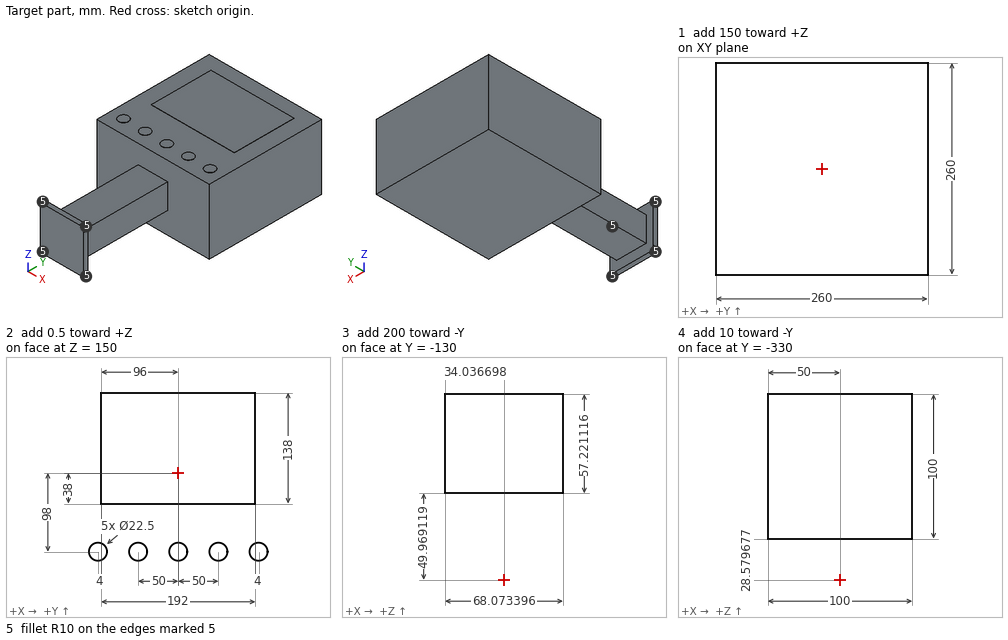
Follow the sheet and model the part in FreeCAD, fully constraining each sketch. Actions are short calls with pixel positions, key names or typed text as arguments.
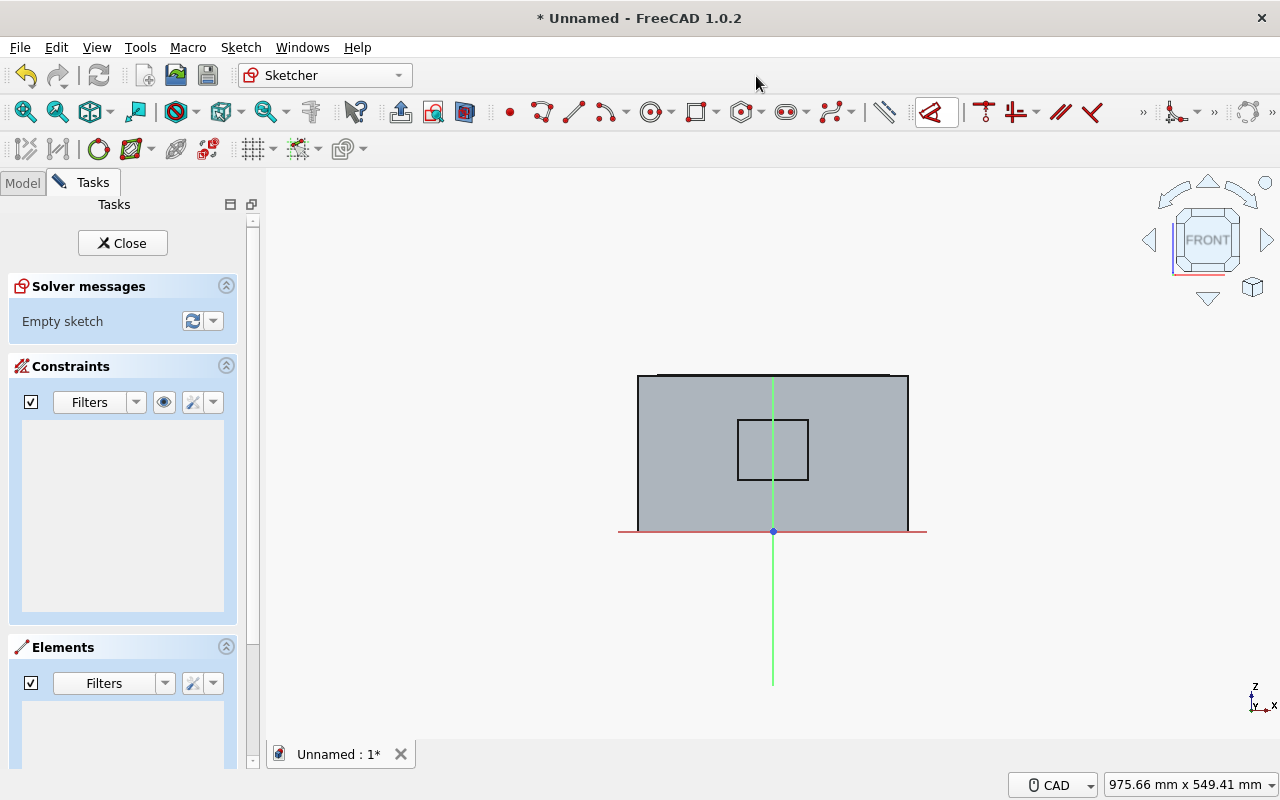
scroll(813, 472, up, 5)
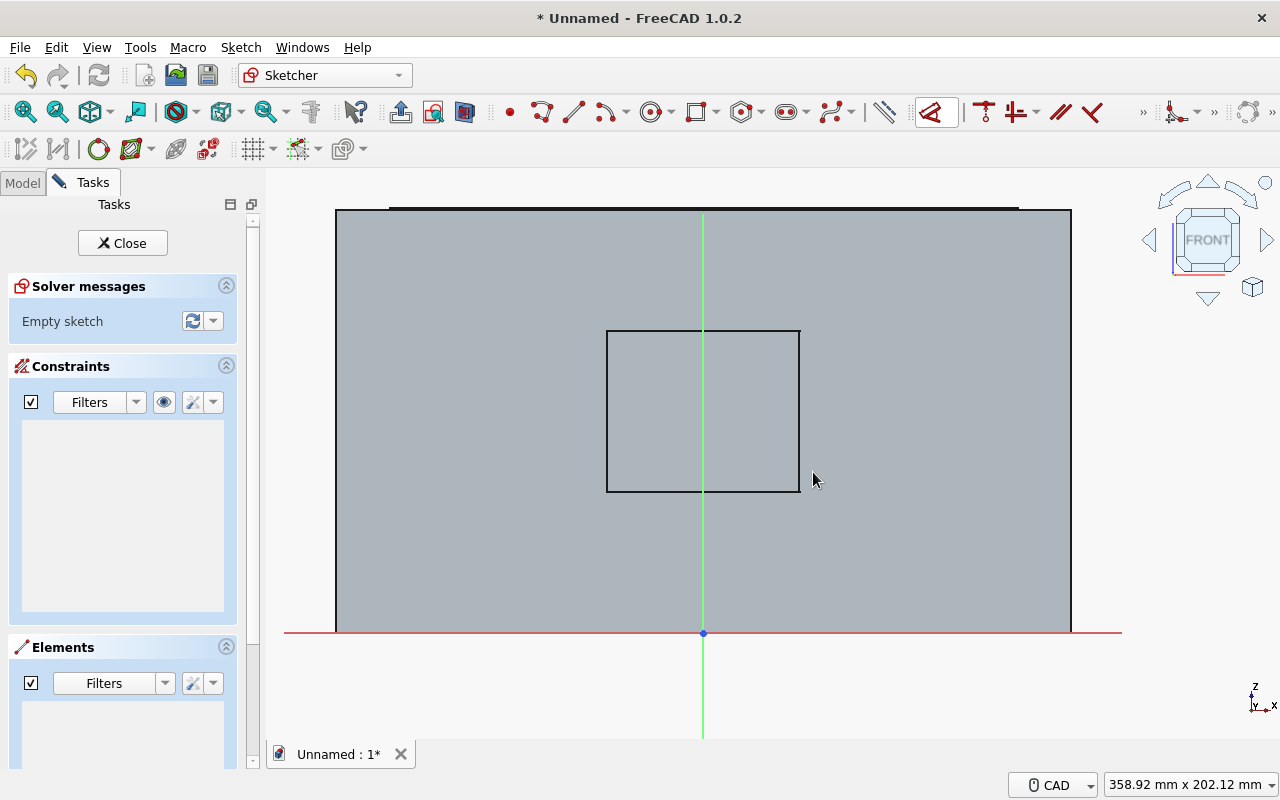
key(g)
key(r)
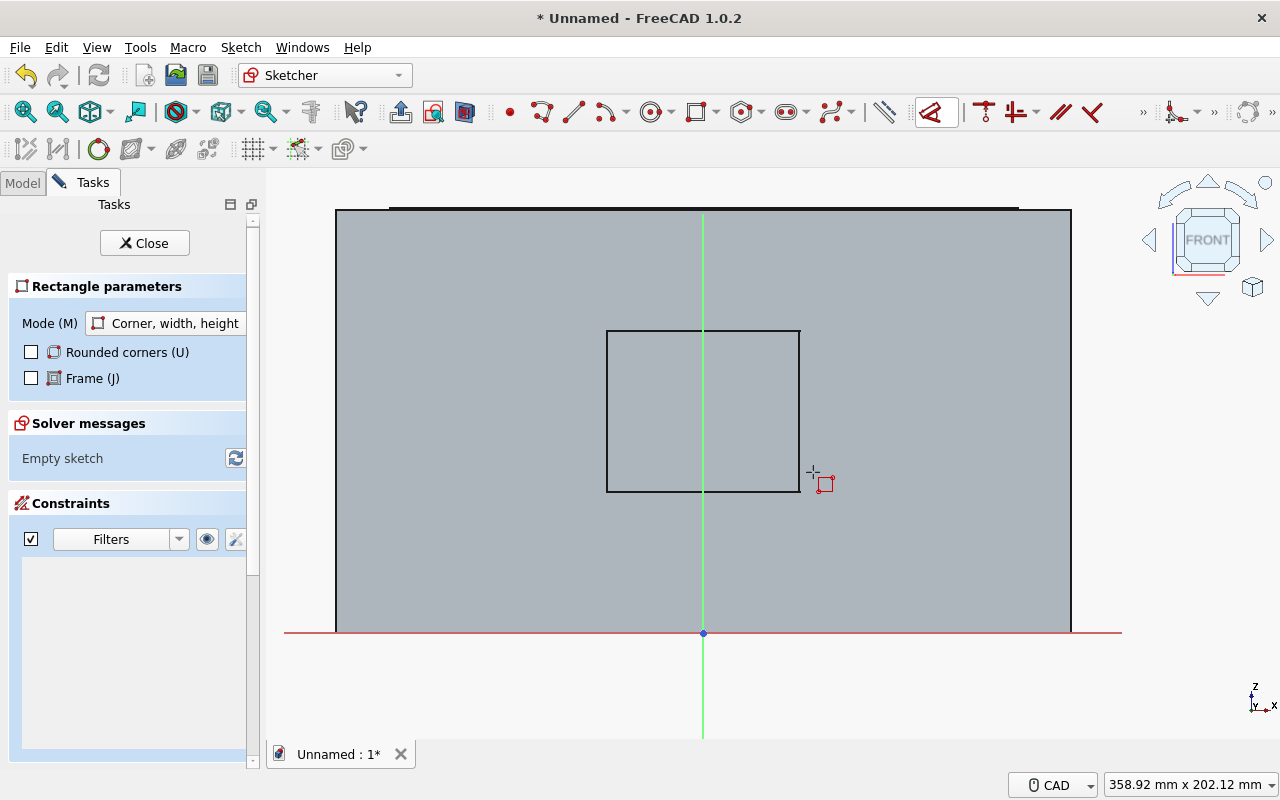
click(562, 270)
move(845, 553)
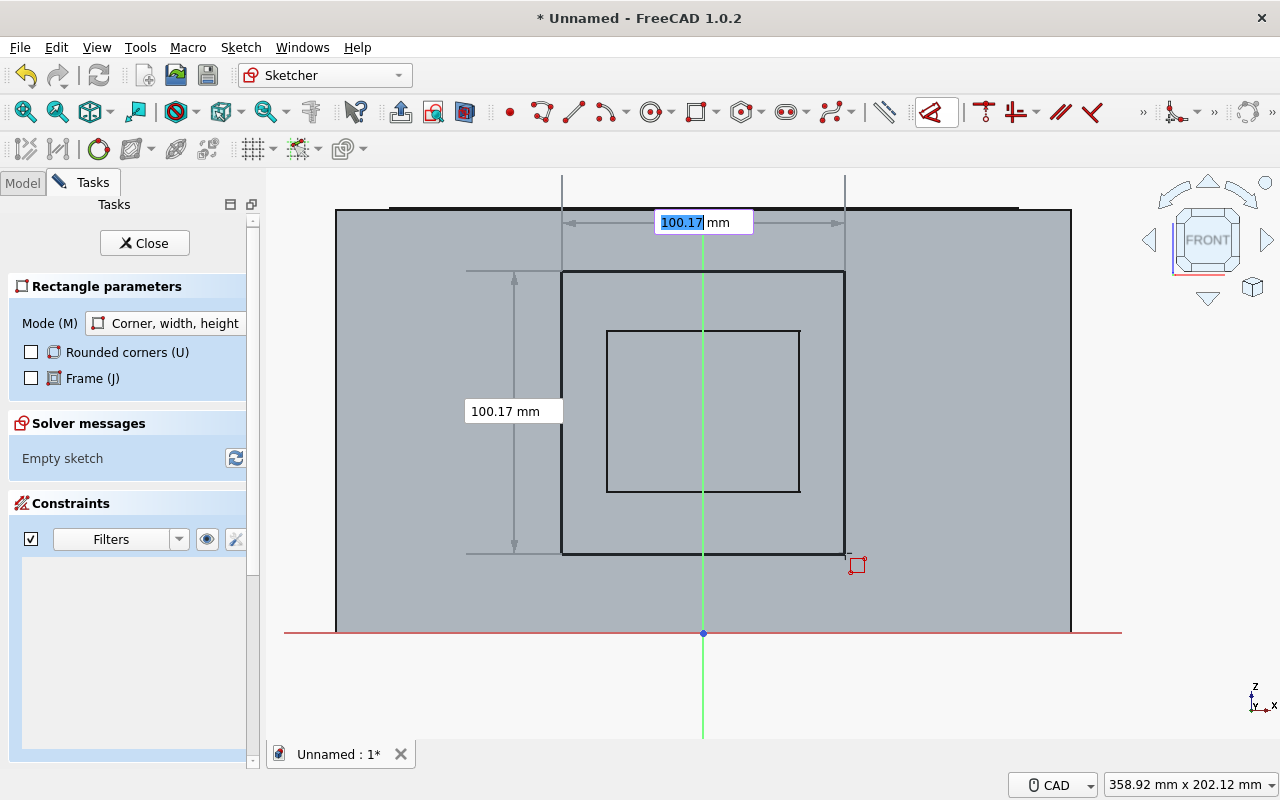
text(100)
key(Tab)
text(100)
key(Return)
key(Escape)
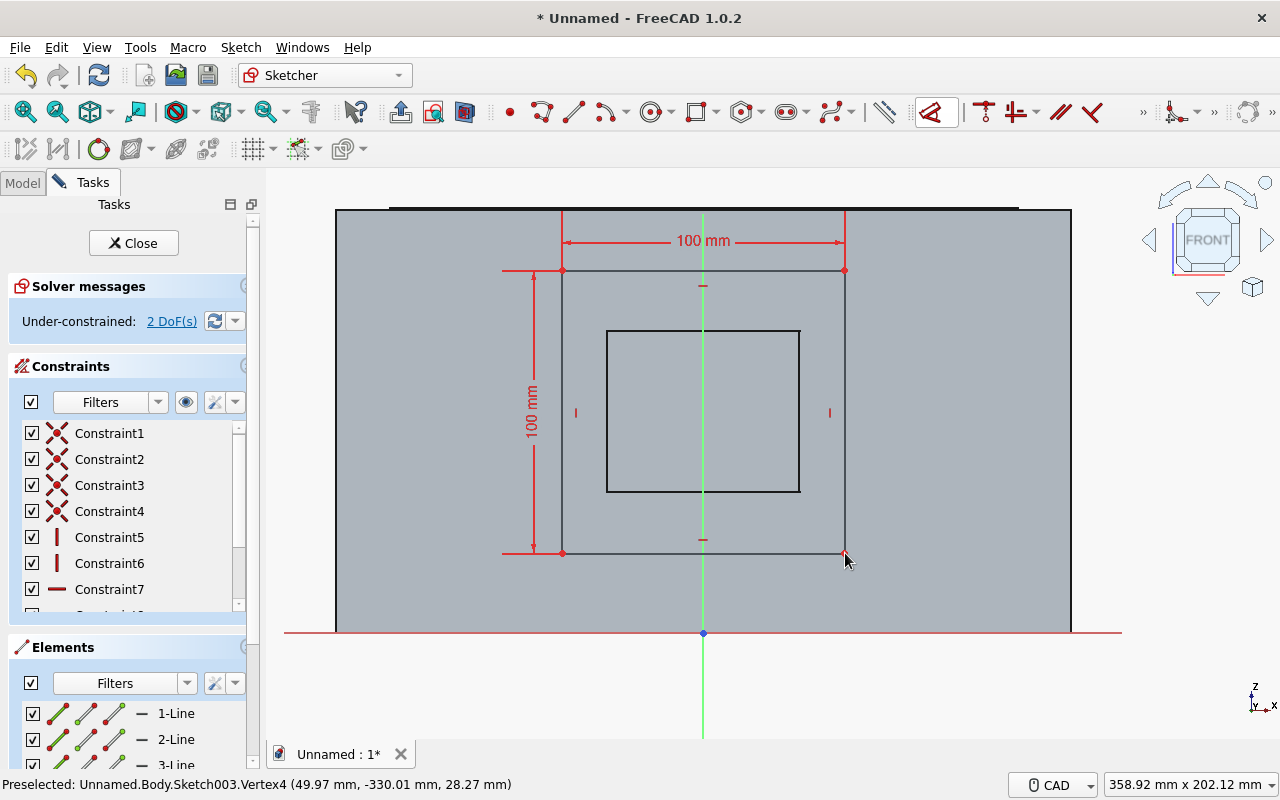
click(562, 271)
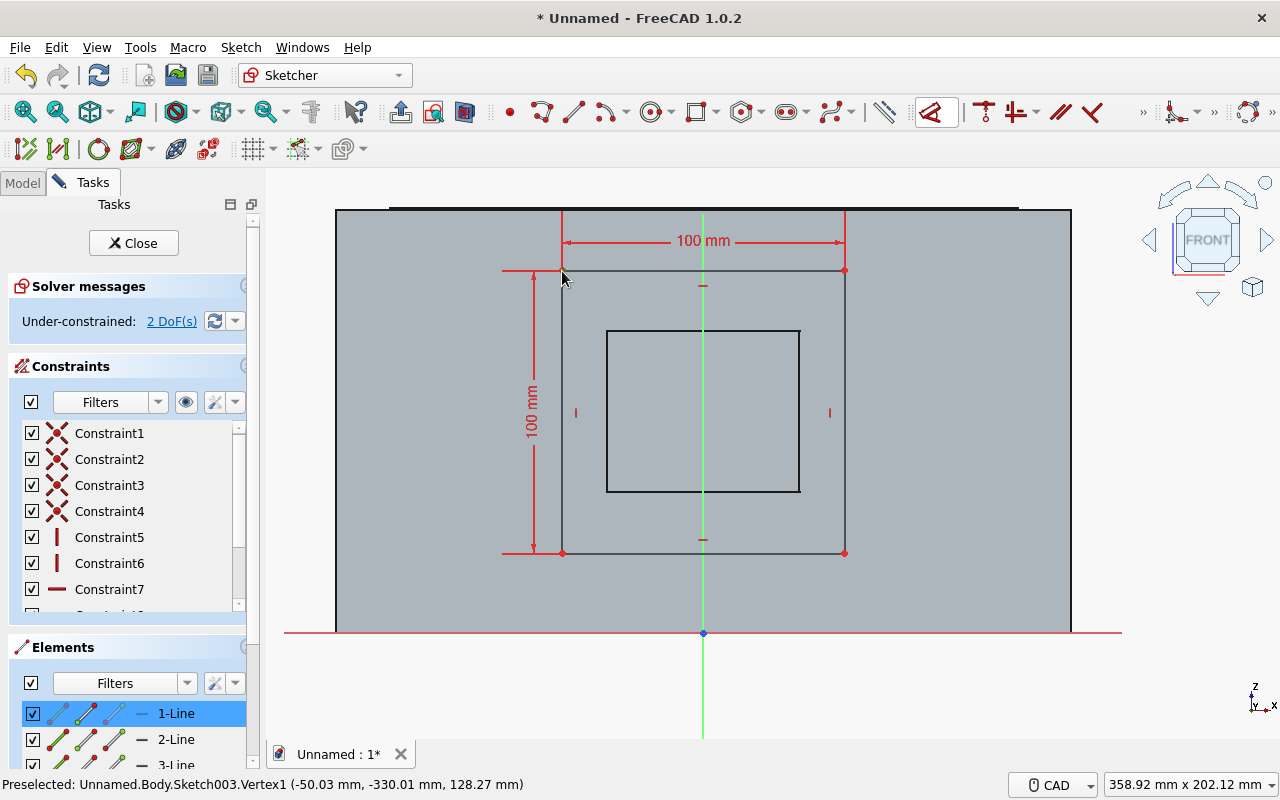
key(l)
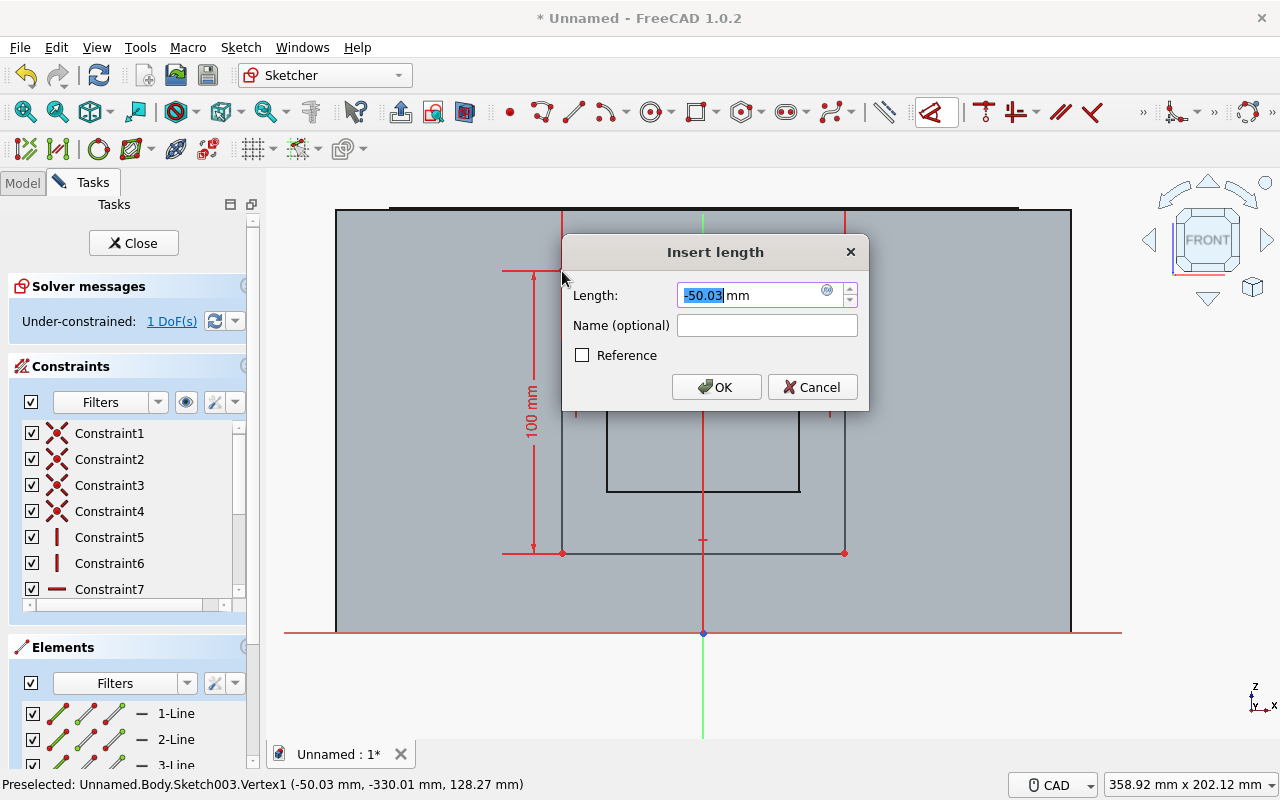
text(-50)
key(Return)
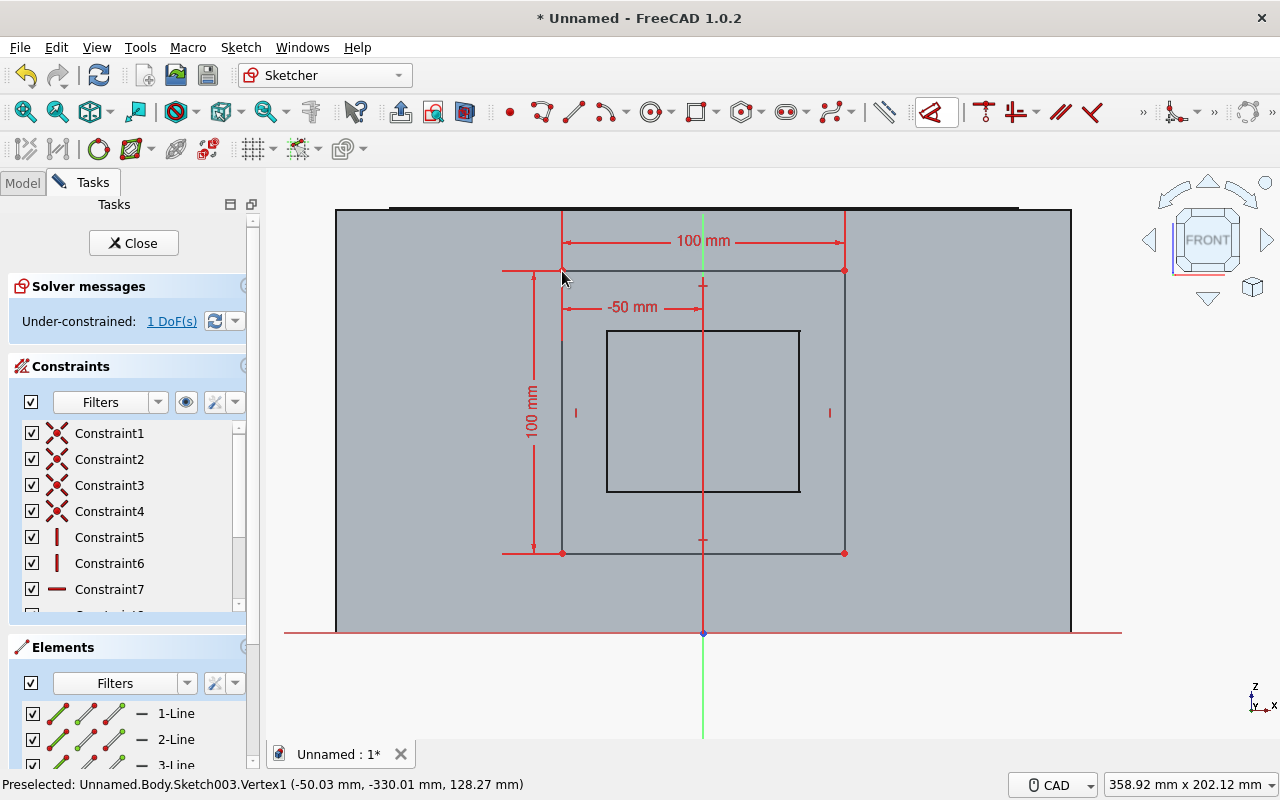
click(562, 554)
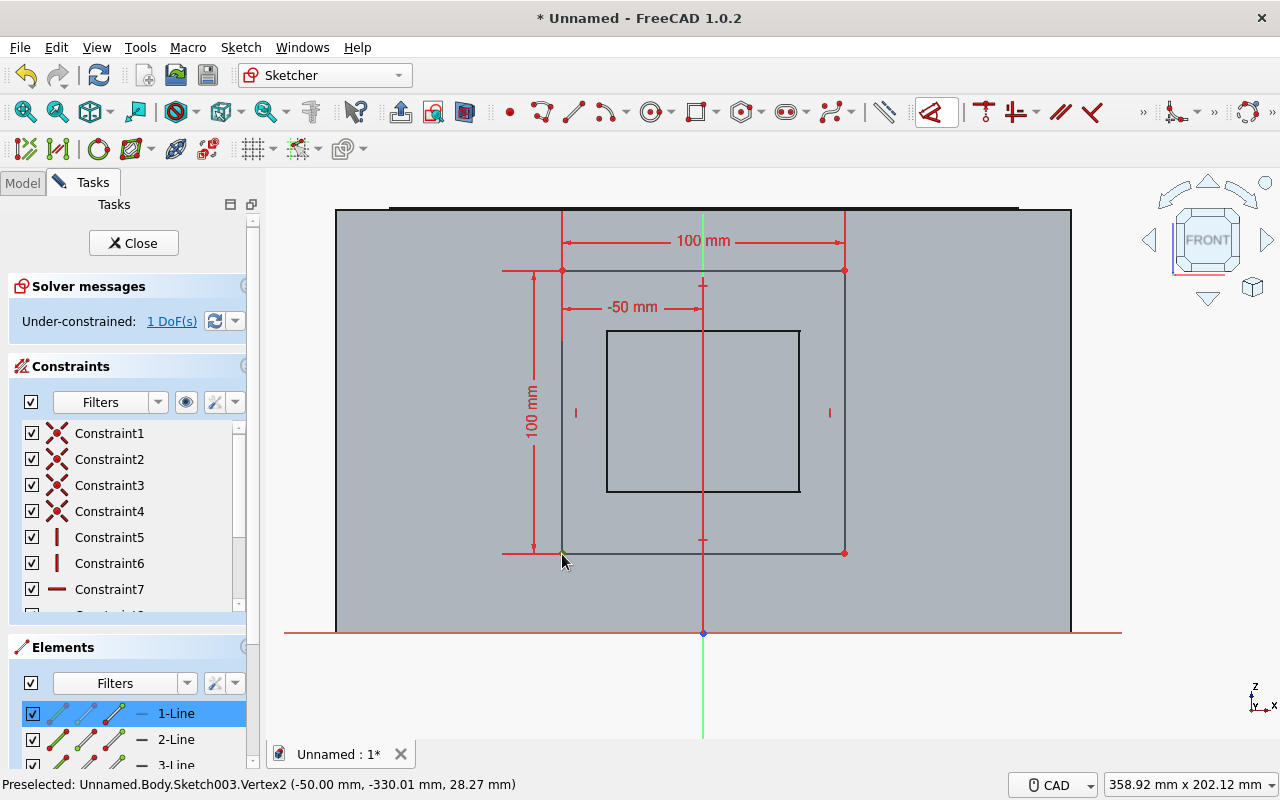
click(952, 112)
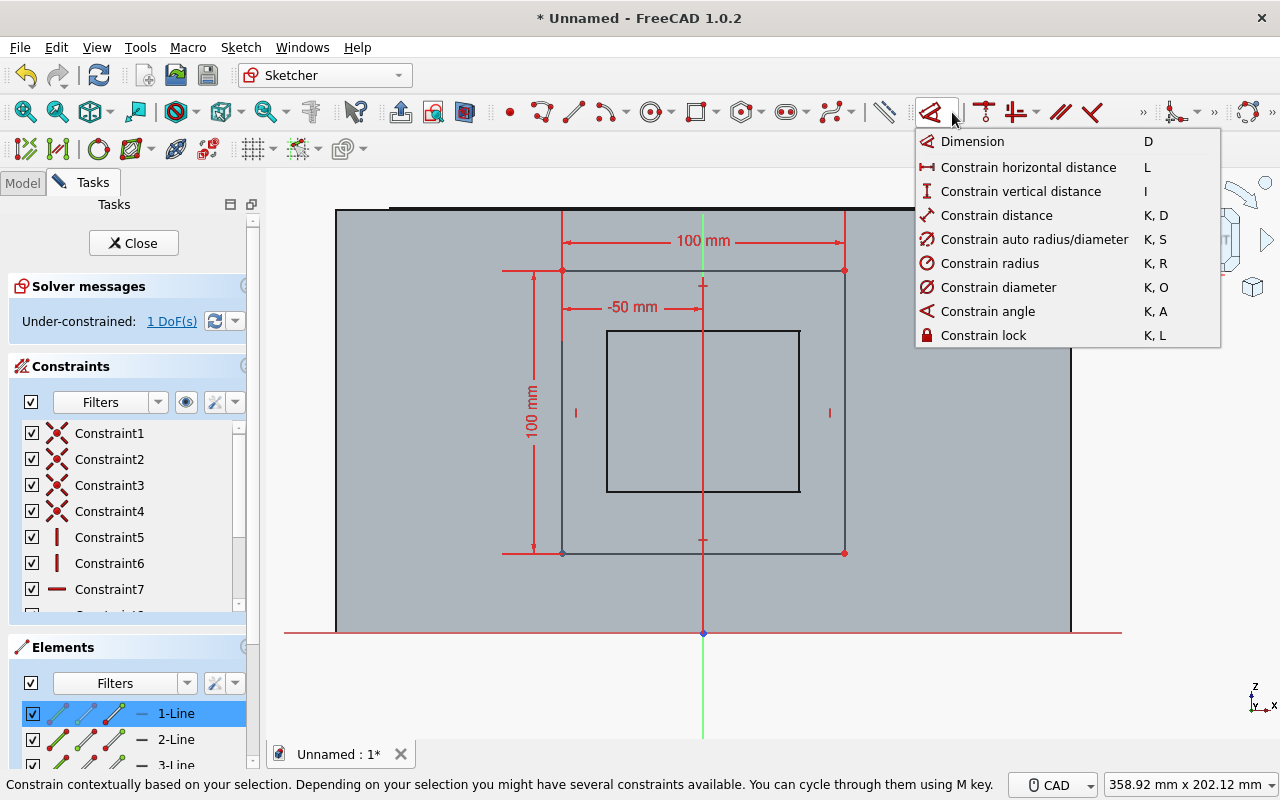
click(1068, 191)